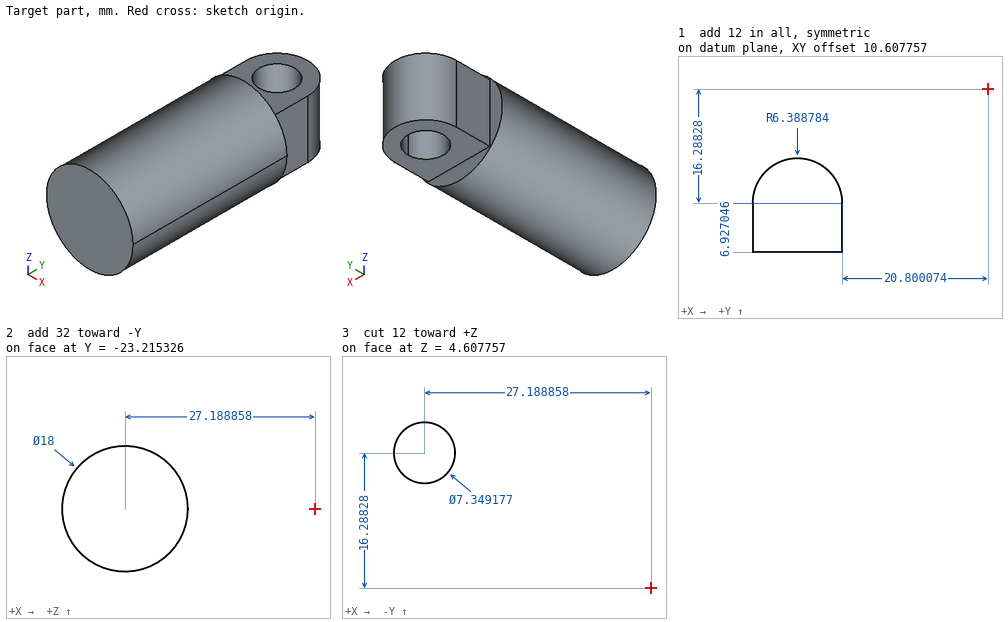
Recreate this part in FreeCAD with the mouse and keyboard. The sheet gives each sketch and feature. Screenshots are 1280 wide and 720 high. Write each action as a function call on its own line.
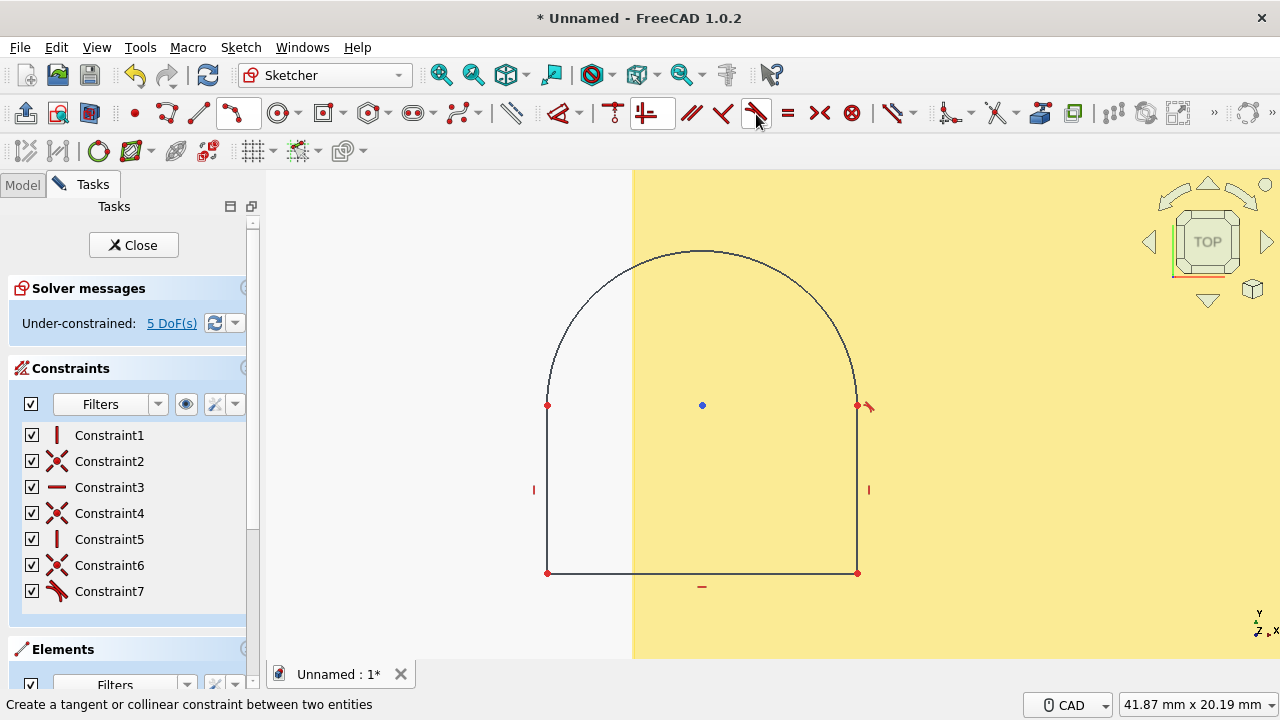
click(547, 524)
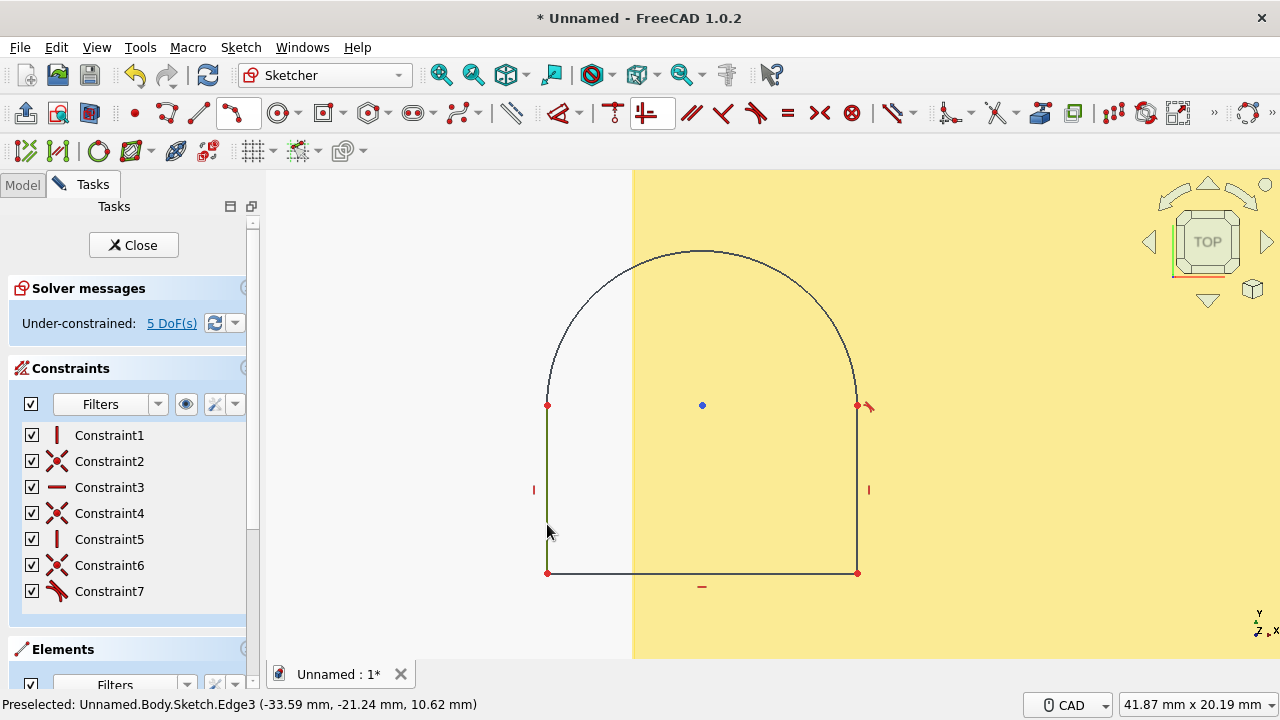
click(793, 281)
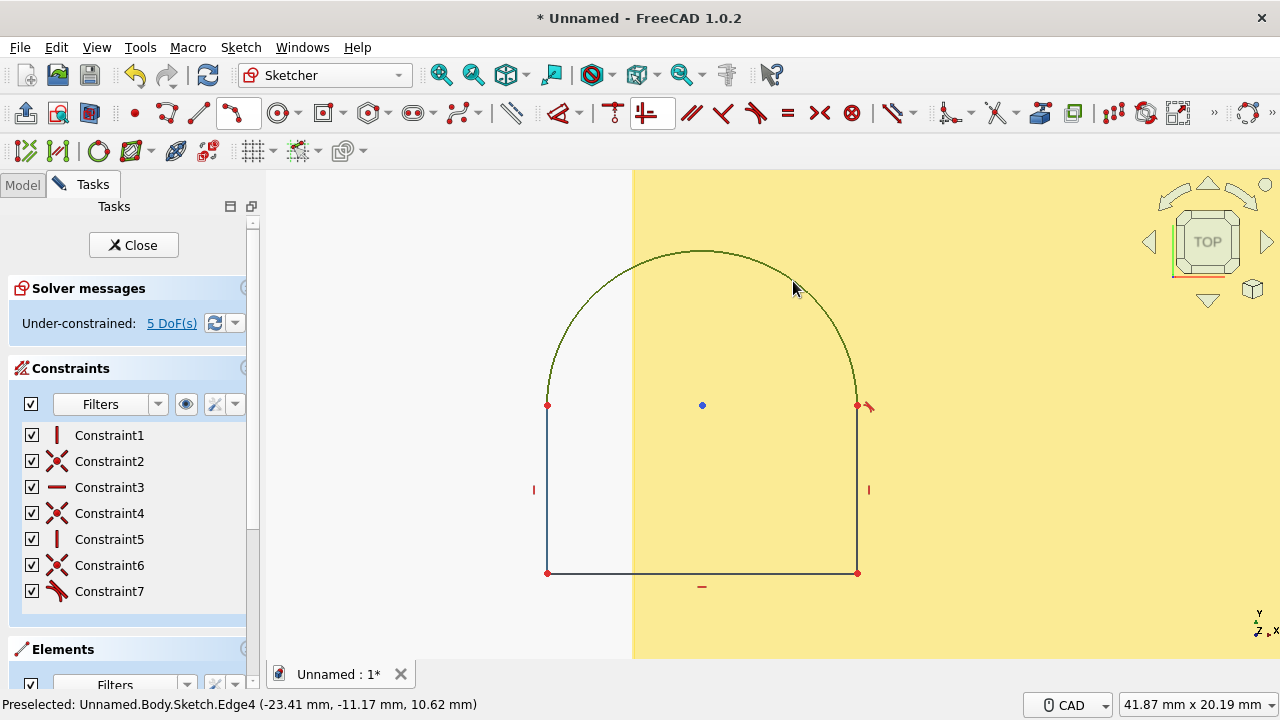
click(756, 114)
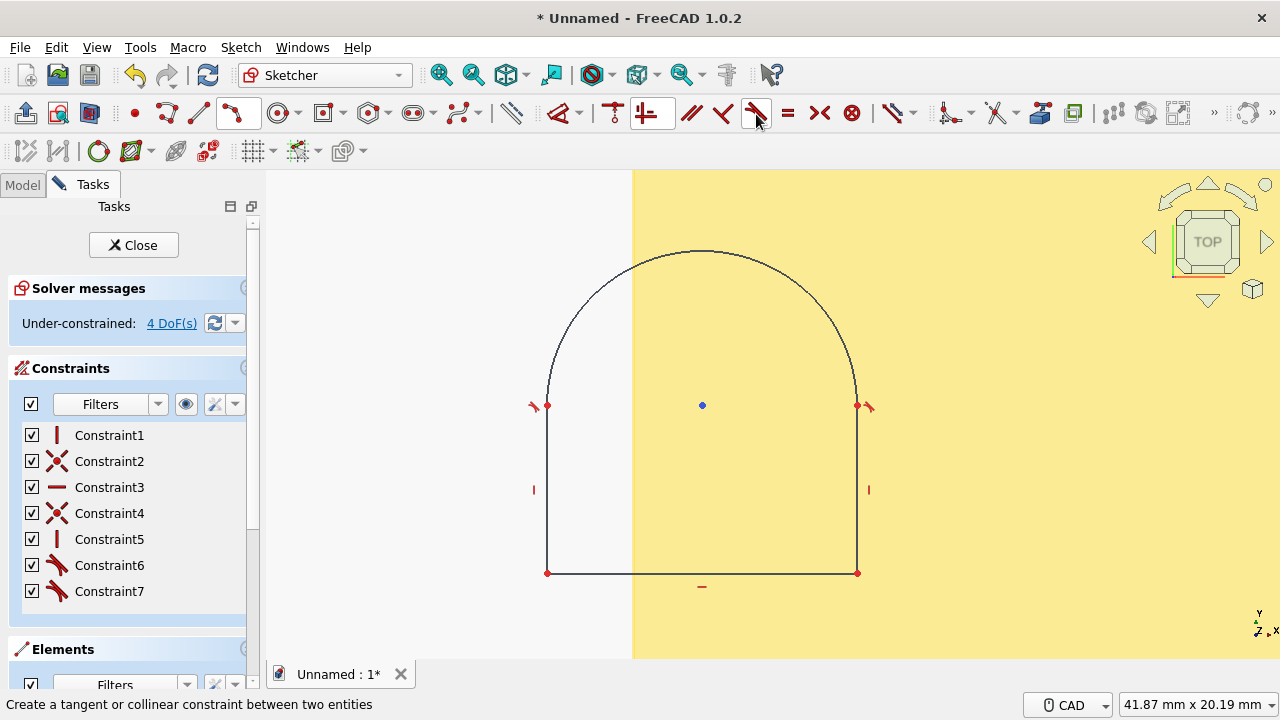
click(558, 114)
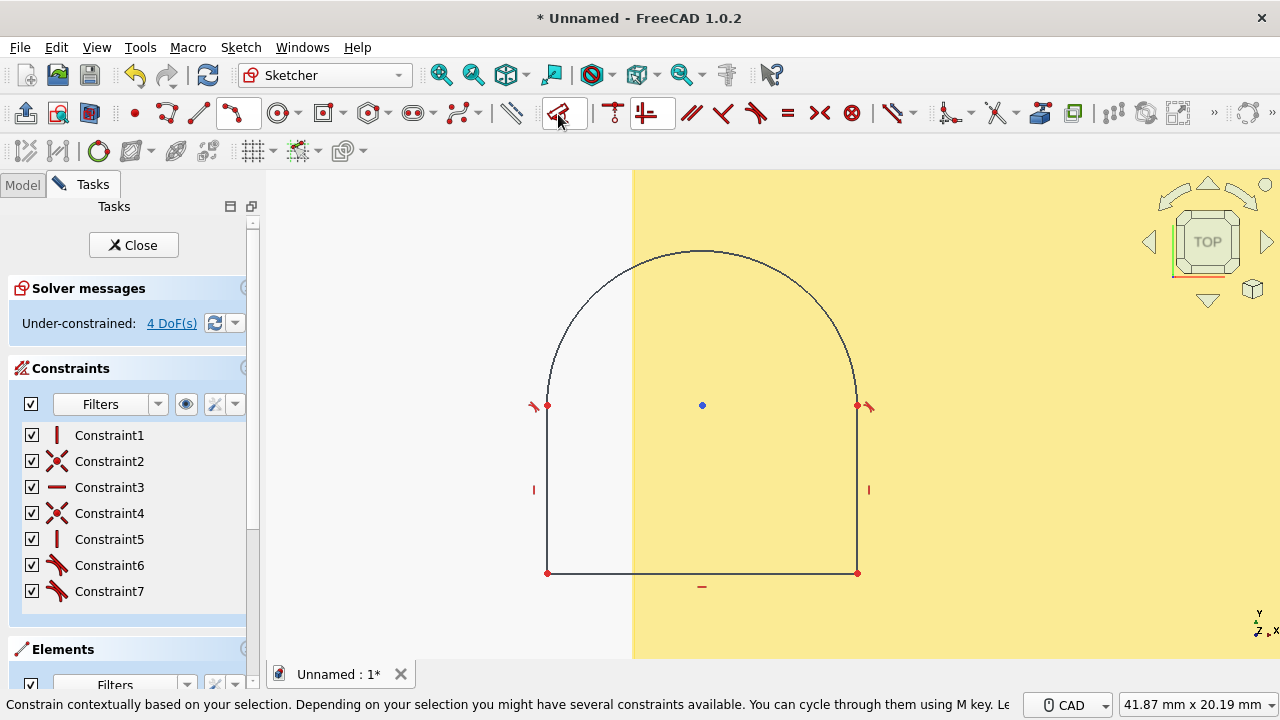
click(793, 281)
click(812, 255)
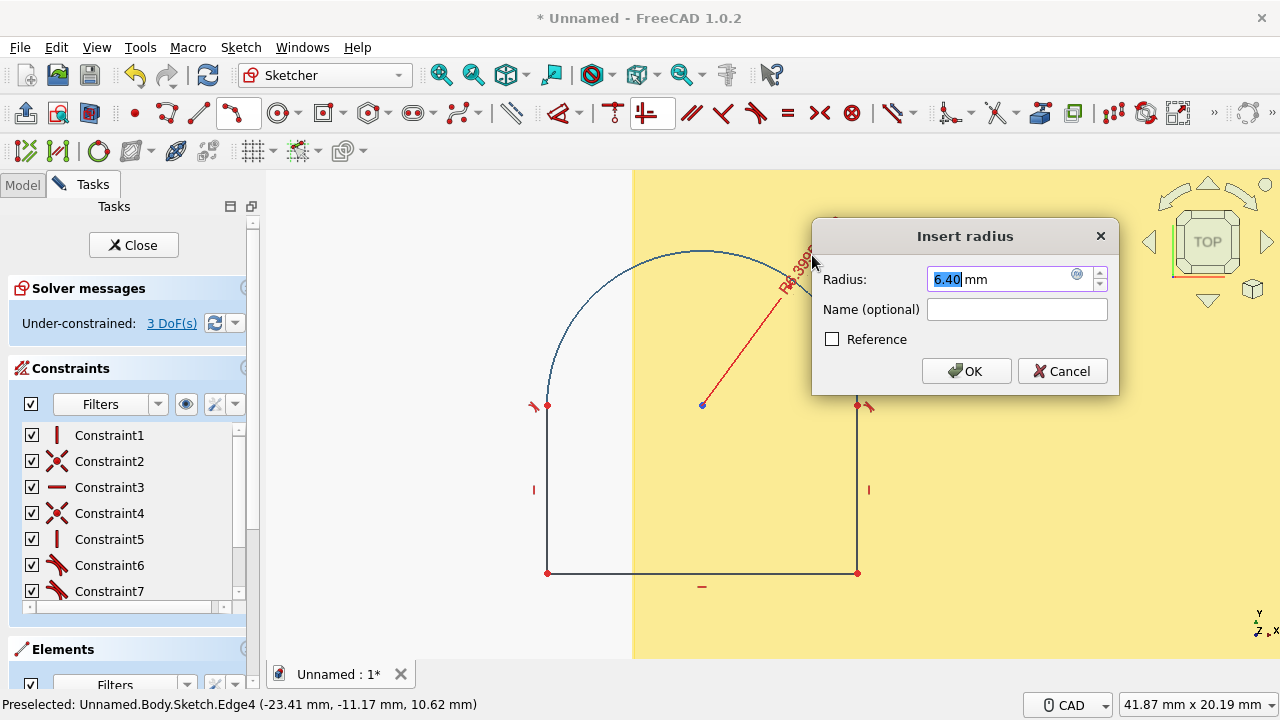
text(6.388784)
key(Return)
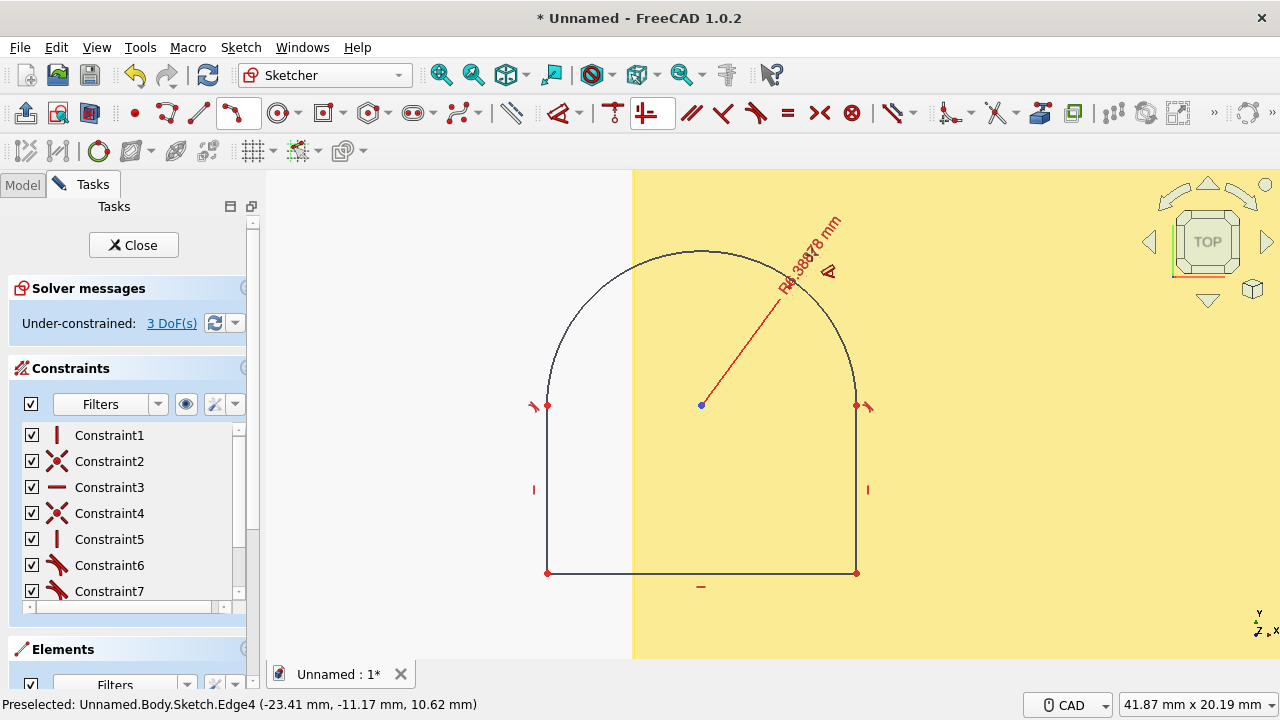
click(856, 456)
click(890, 490)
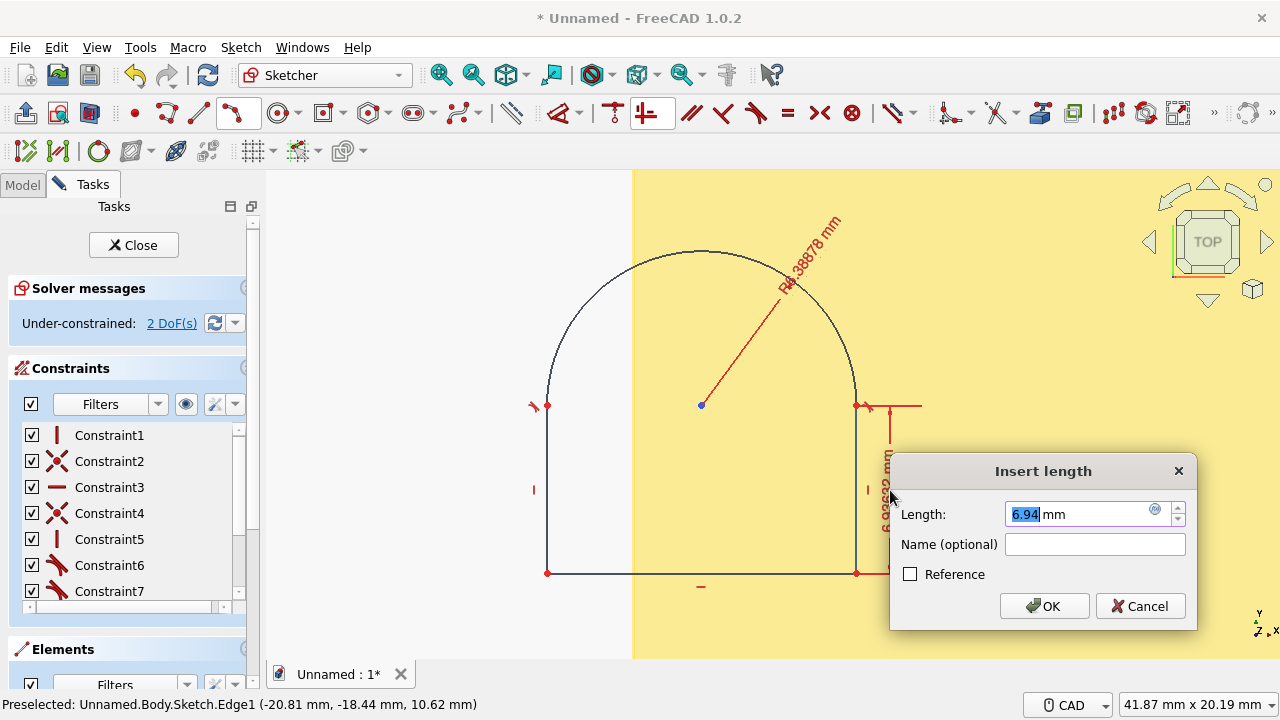
text(6.927046)
key(Return)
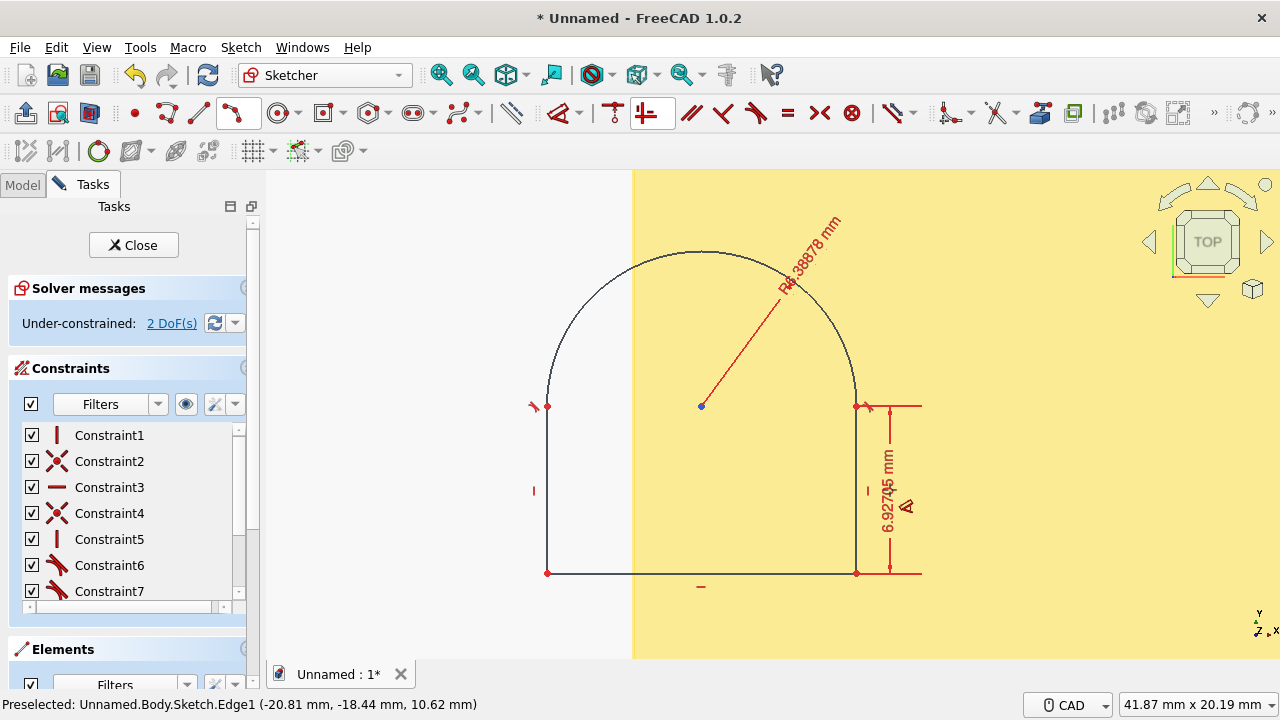
click(856, 406)
click(822, 350)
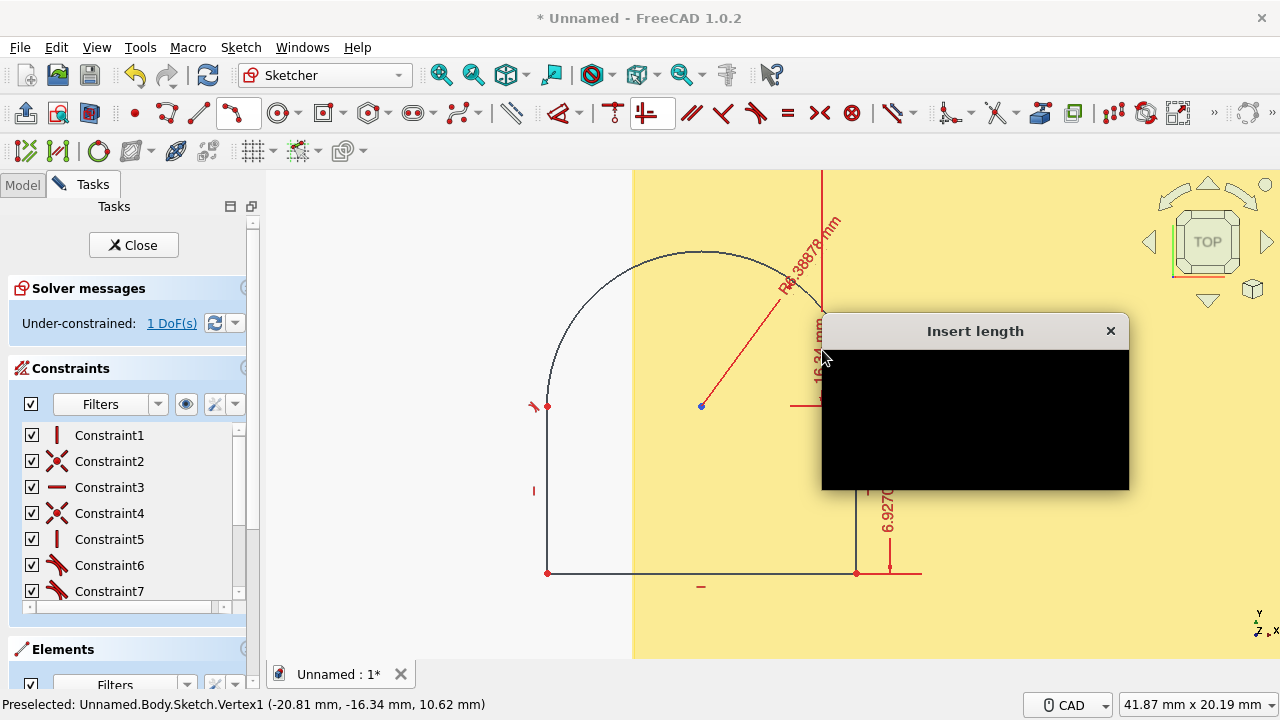
text(16.28828)
key(Return)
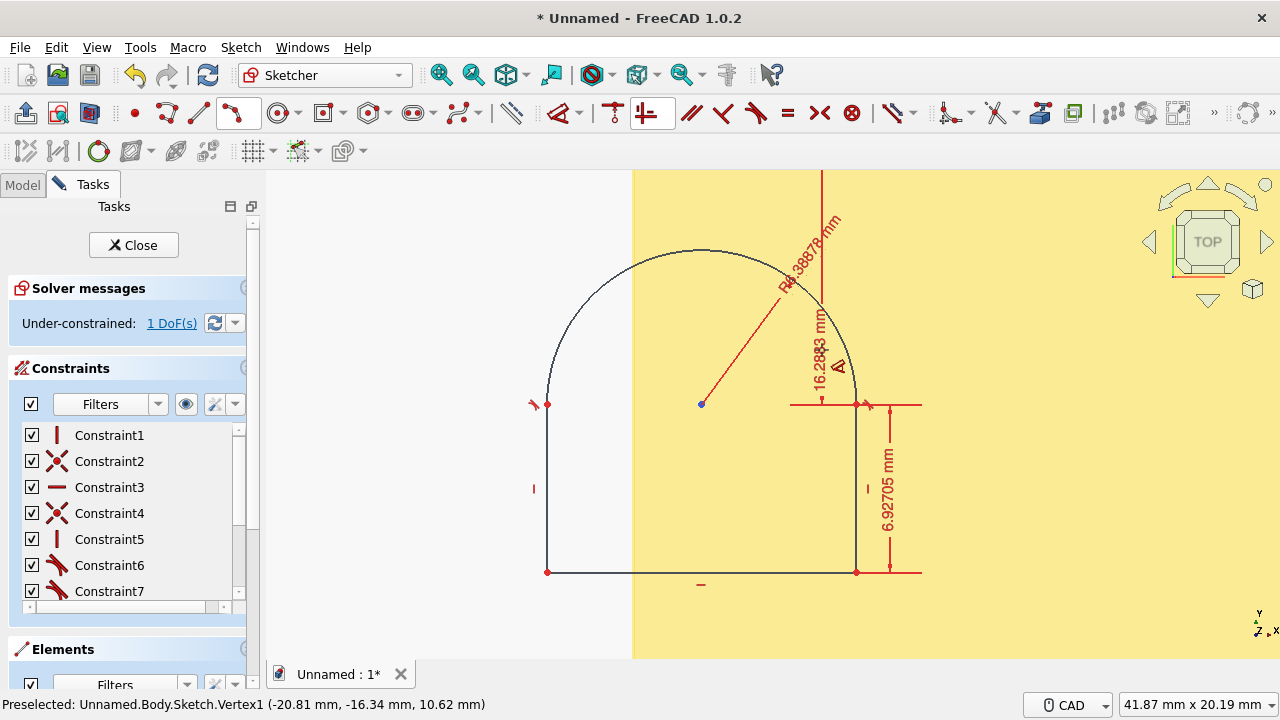
click(856, 405)
click(986, 439)